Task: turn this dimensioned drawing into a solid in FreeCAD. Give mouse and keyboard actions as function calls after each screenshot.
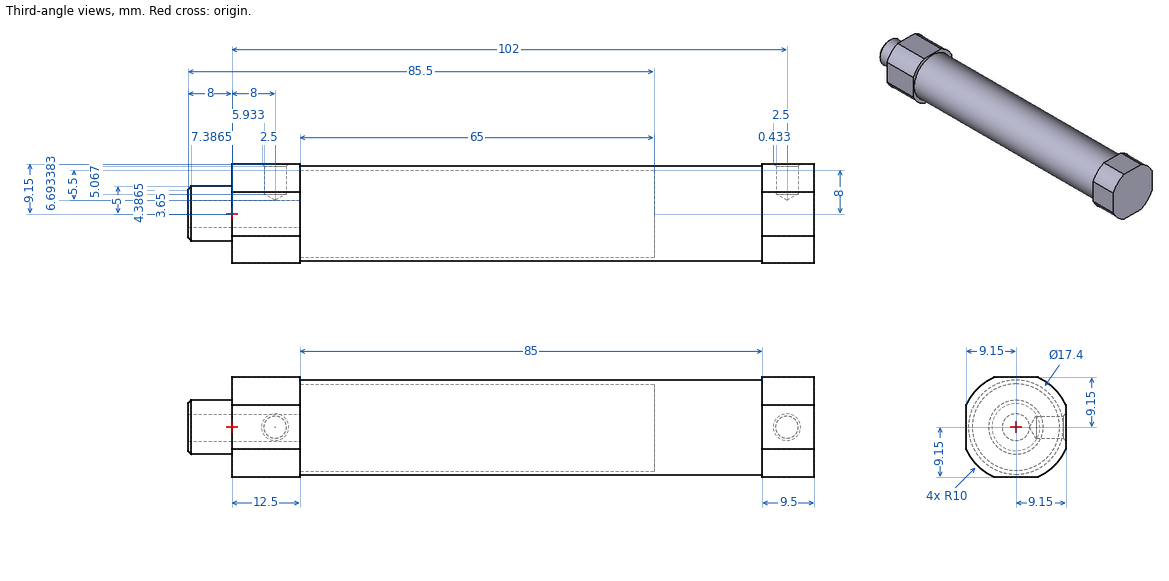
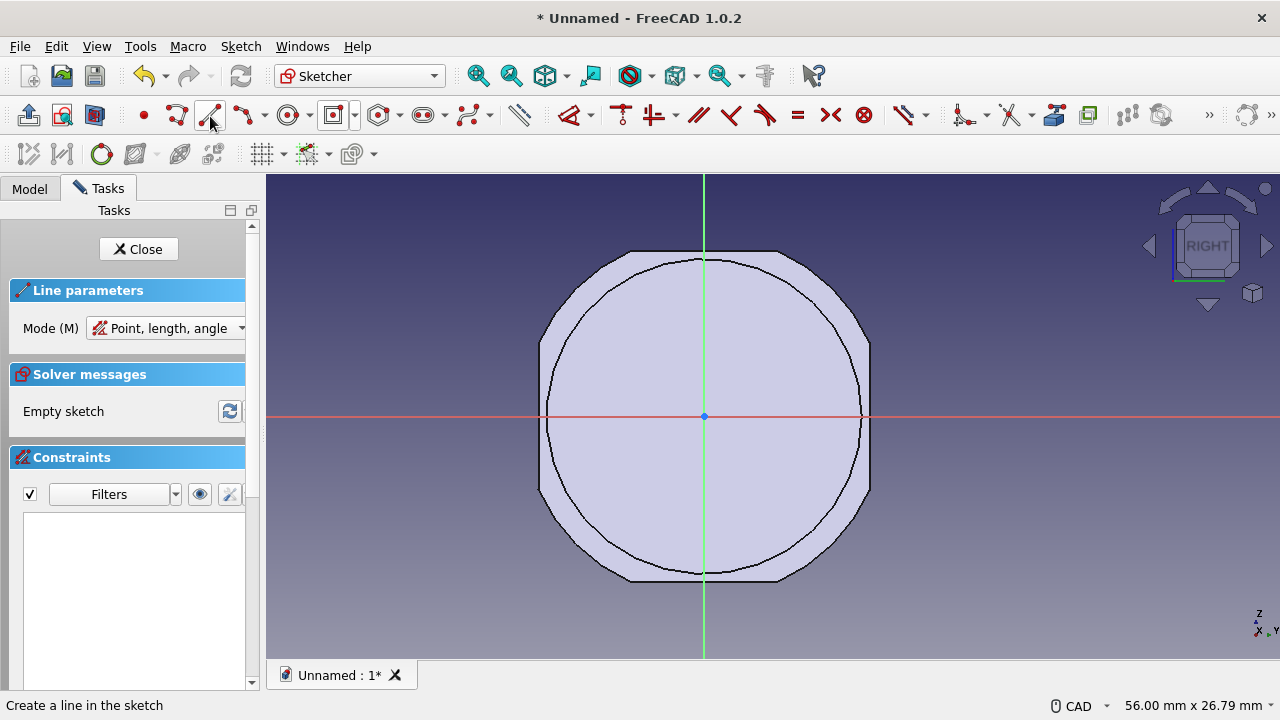
click(539, 343)
click(539, 490)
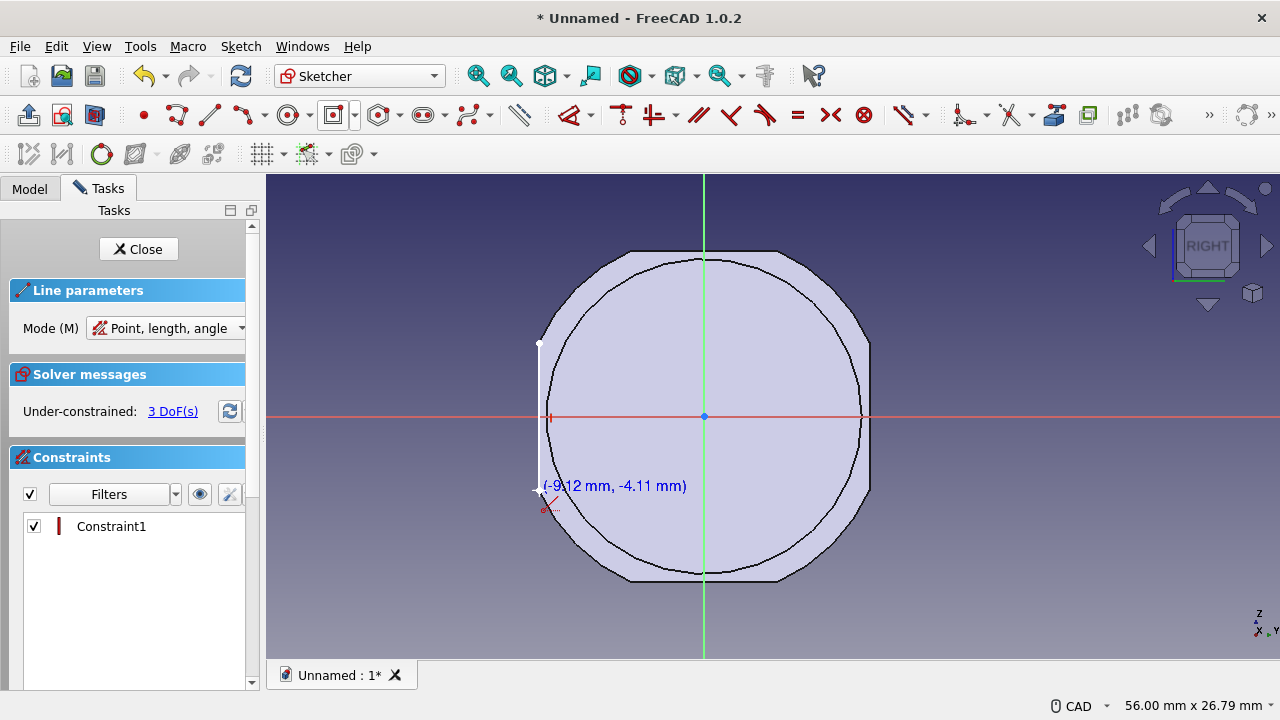
click(631, 582)
click(777, 582)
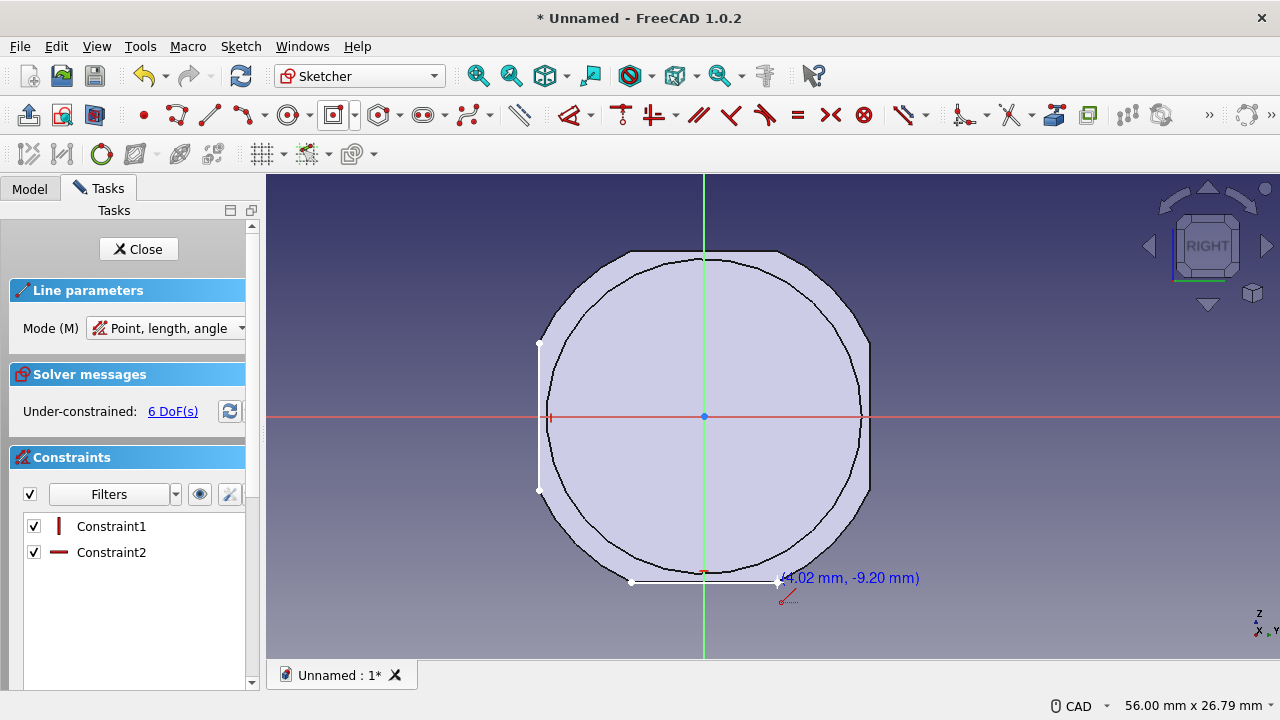
click(870, 490)
click(870, 343)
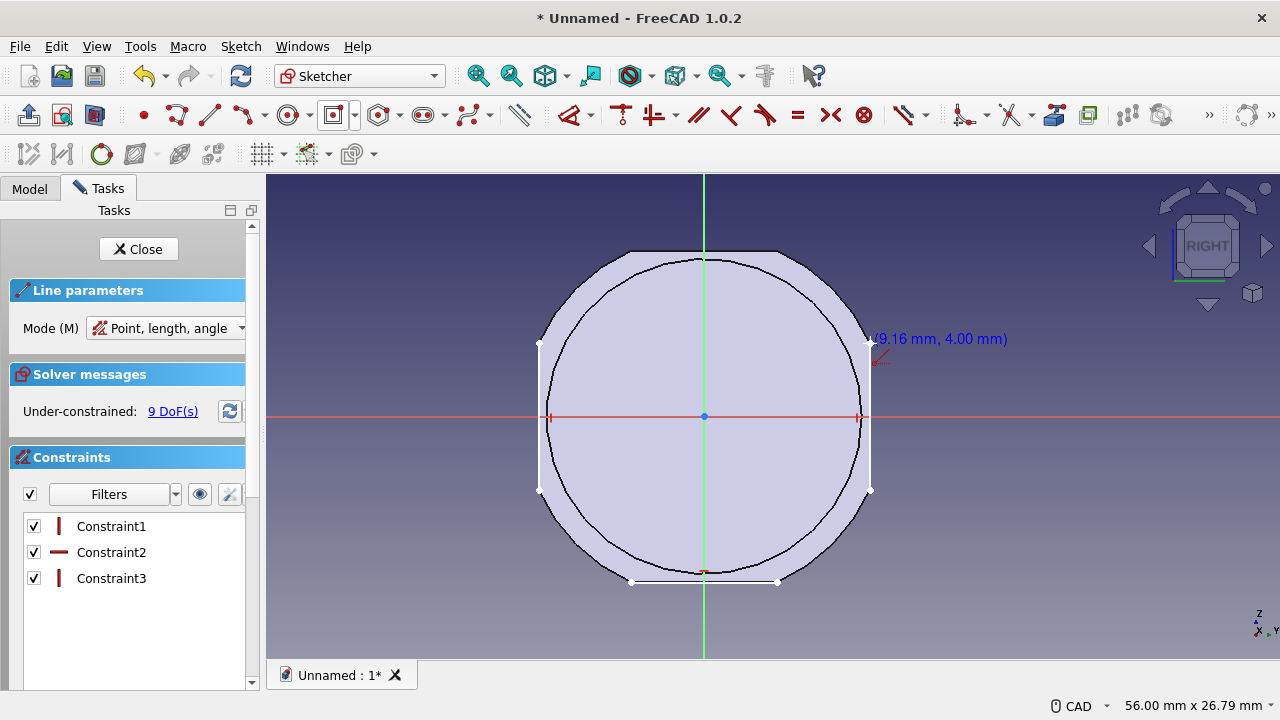
click(777, 251)
click(631, 251)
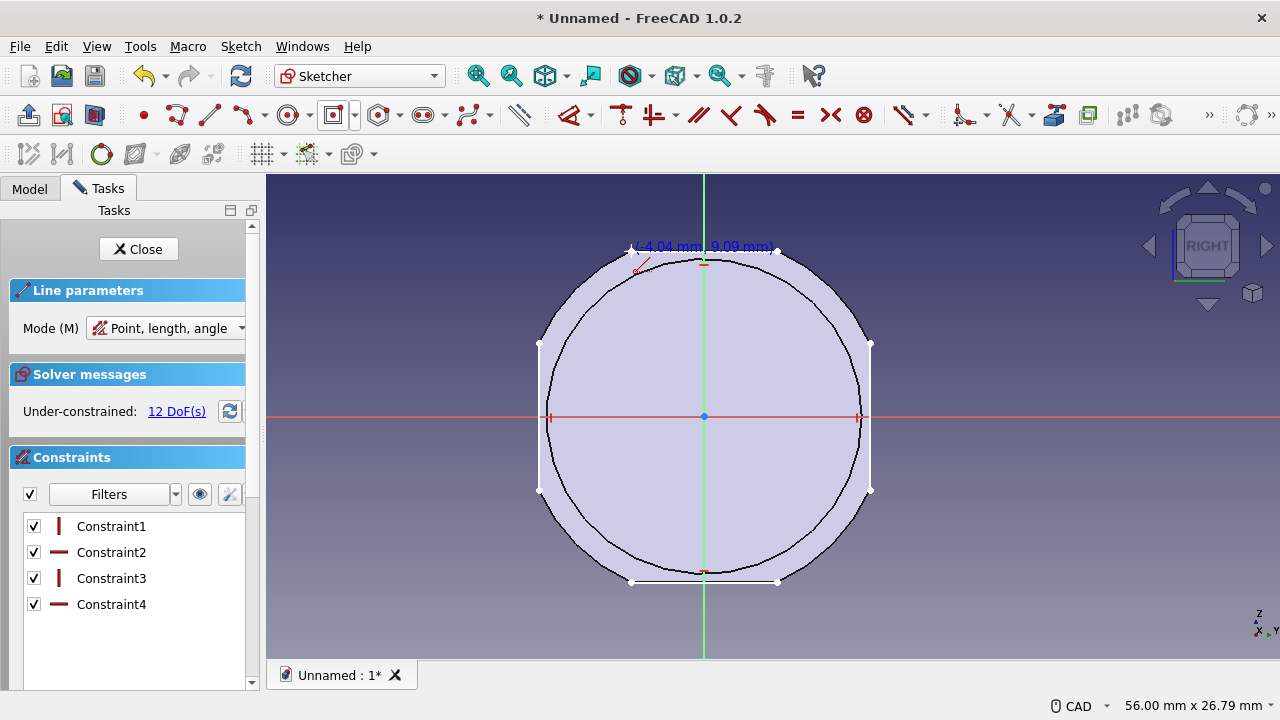
click(242, 116)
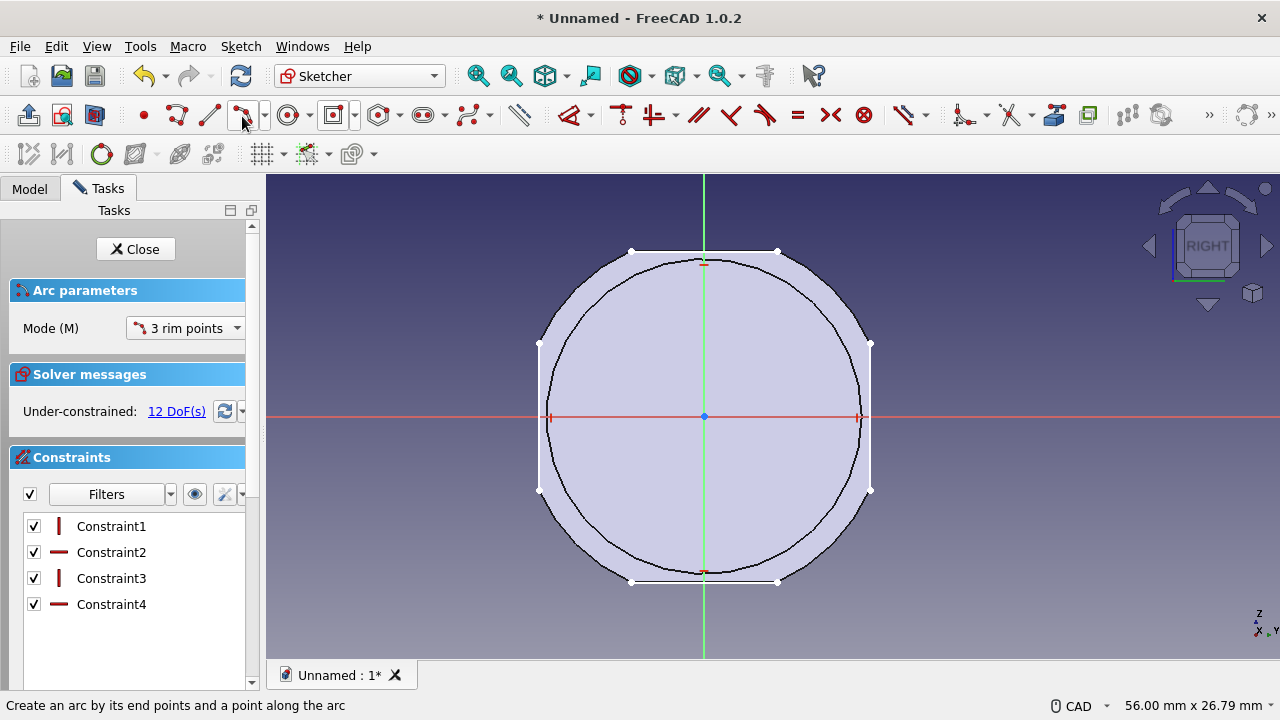
click(539, 491)
click(631, 583)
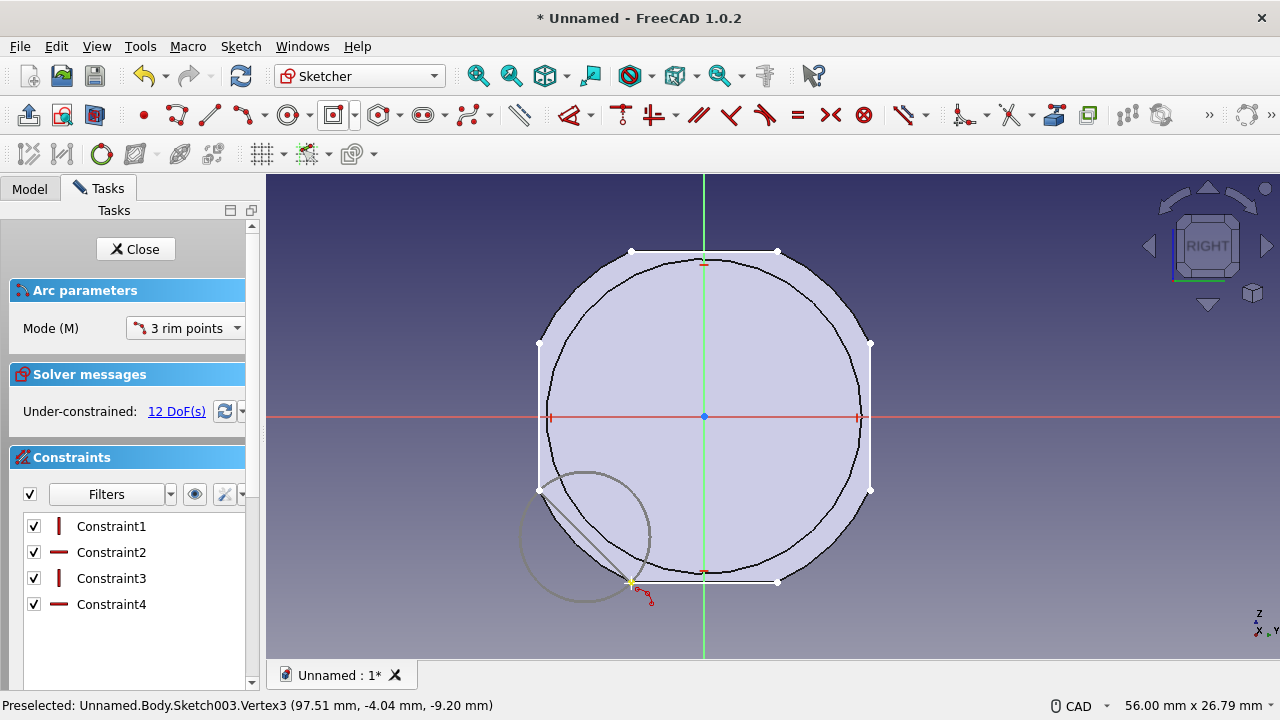
scroll(576, 545, up, 2)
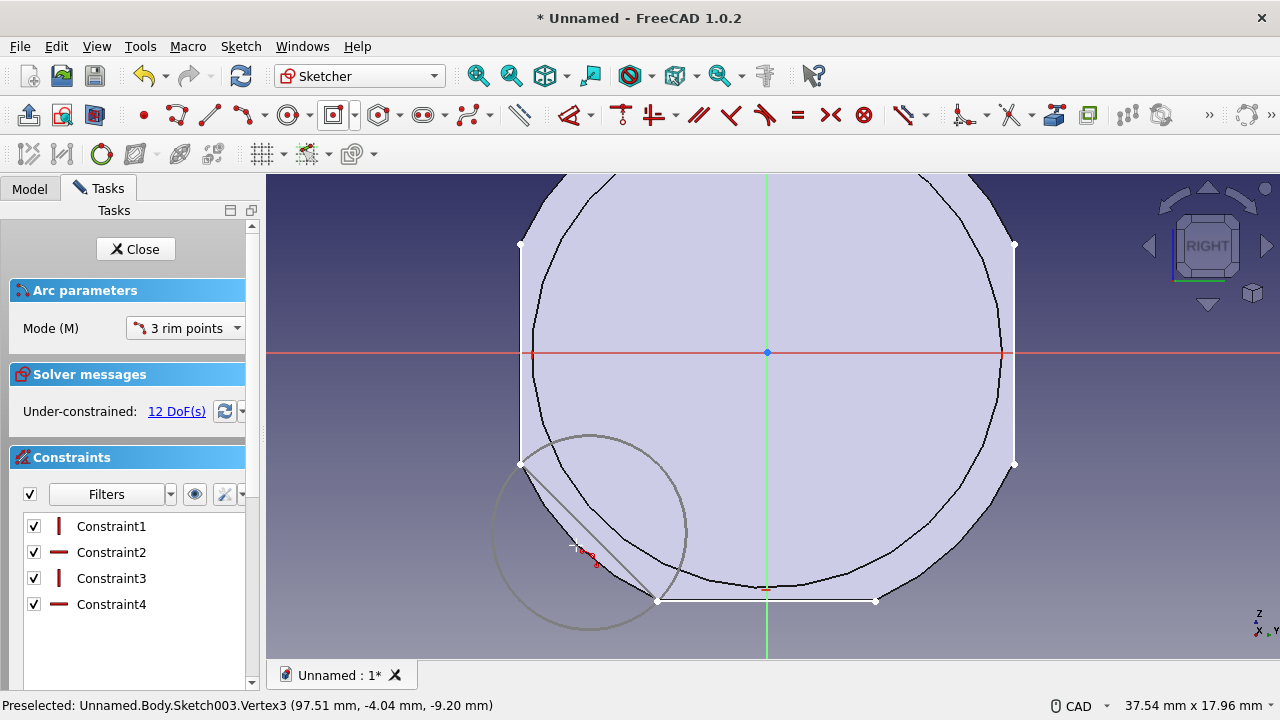
click(576, 544)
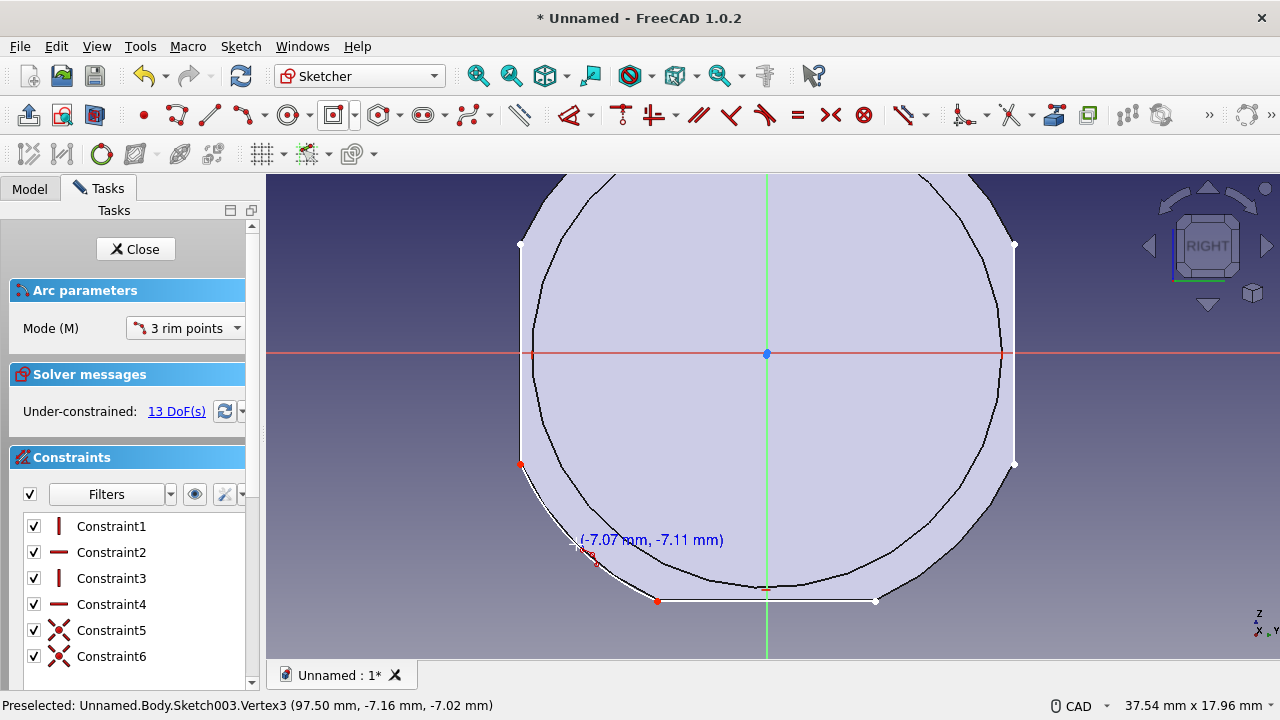
click(876, 601)
click(1014, 464)
click(958, 544)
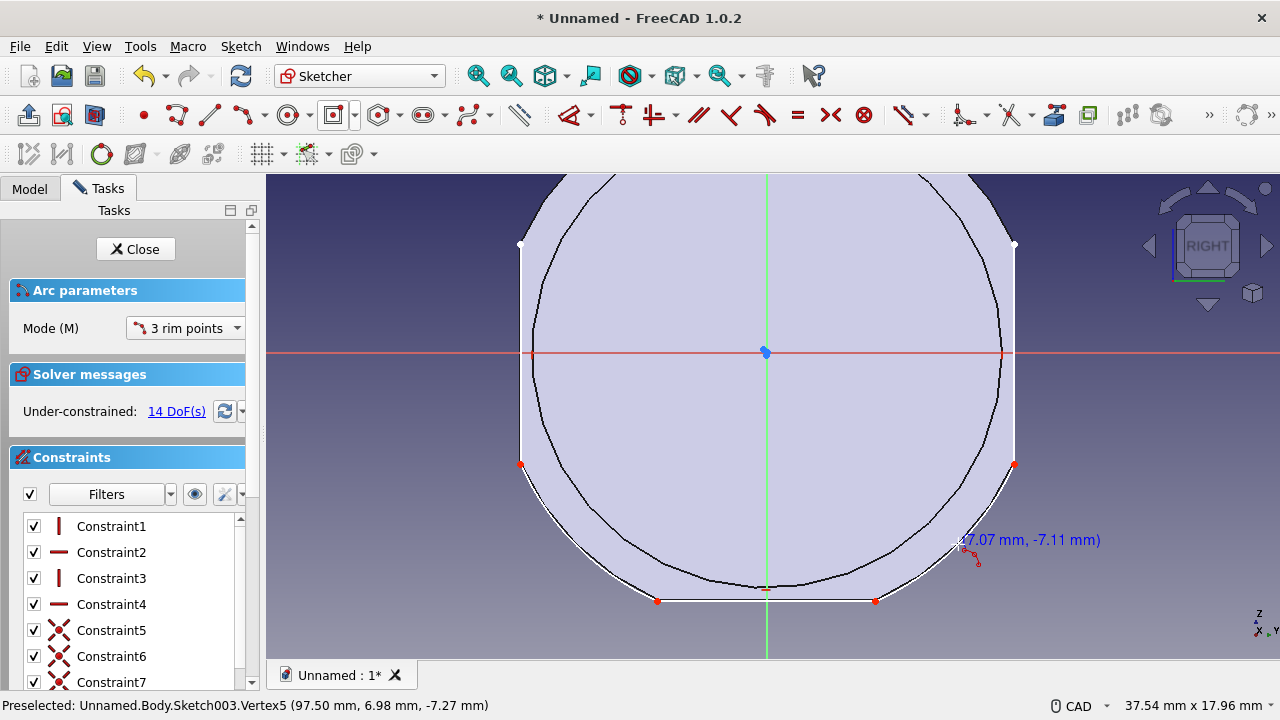
click(1014, 245)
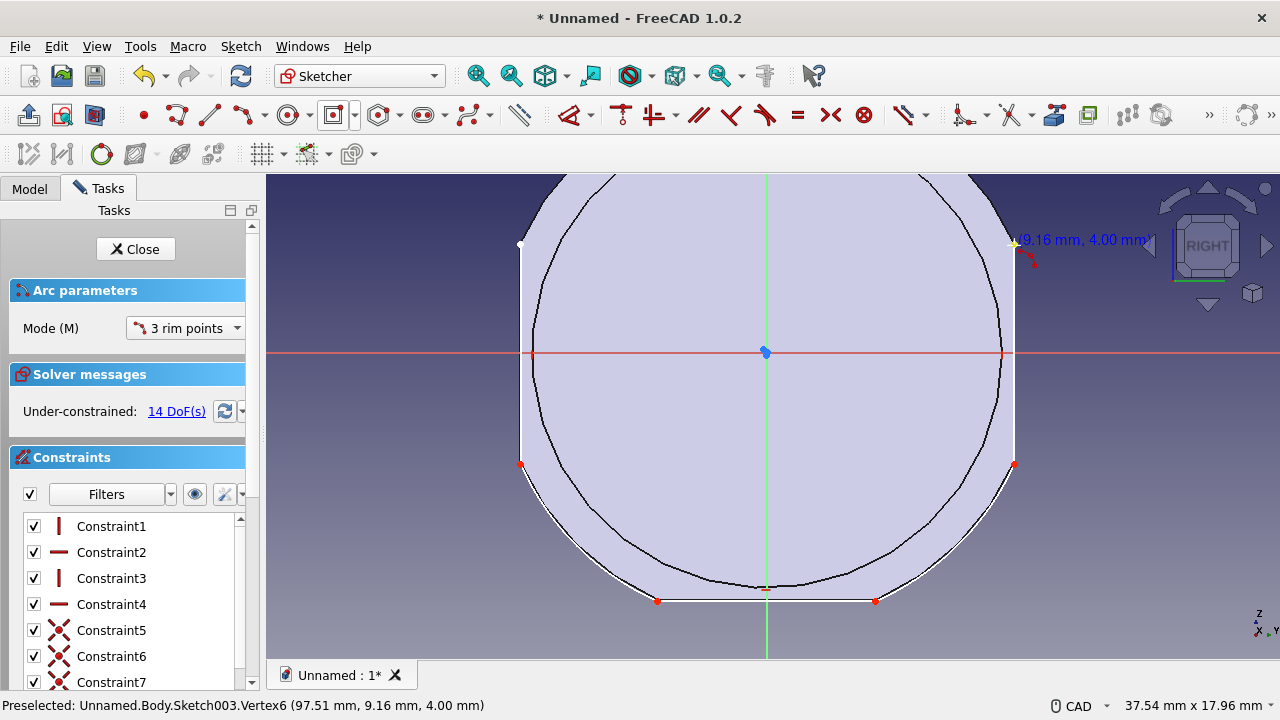
scroll(577, 546, down, 2)